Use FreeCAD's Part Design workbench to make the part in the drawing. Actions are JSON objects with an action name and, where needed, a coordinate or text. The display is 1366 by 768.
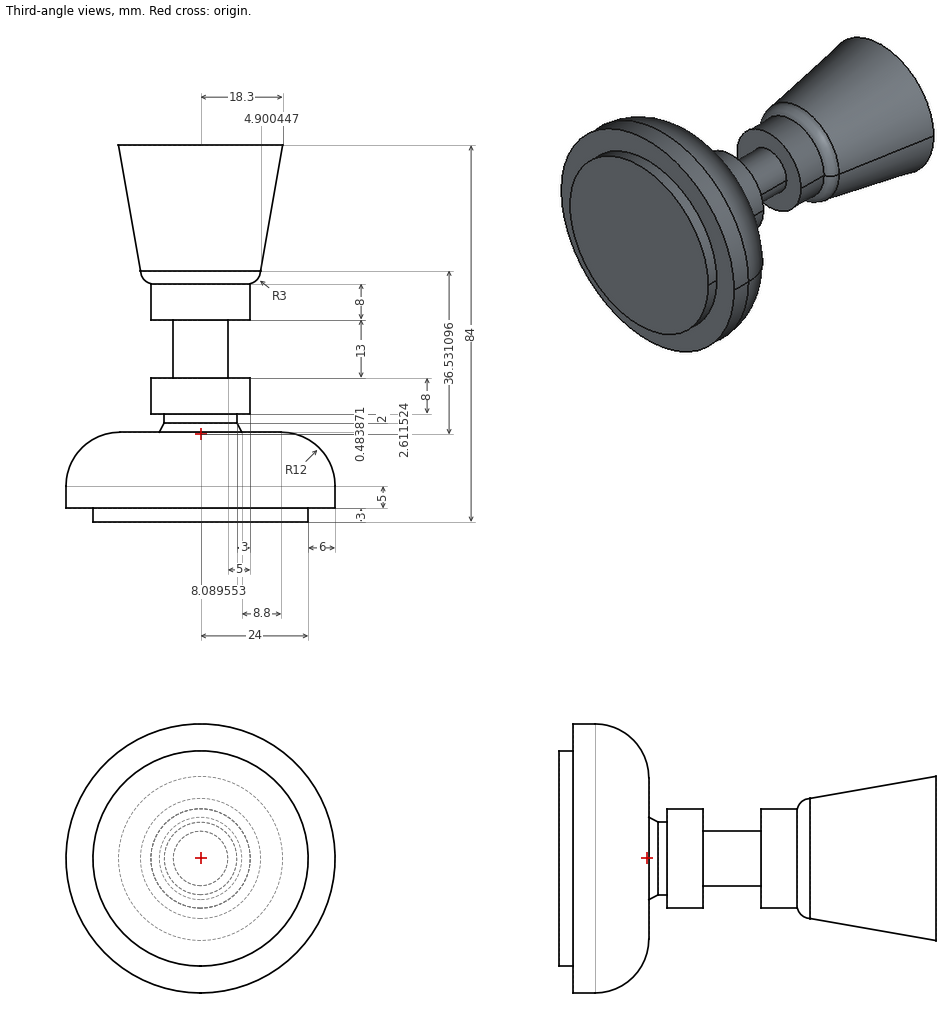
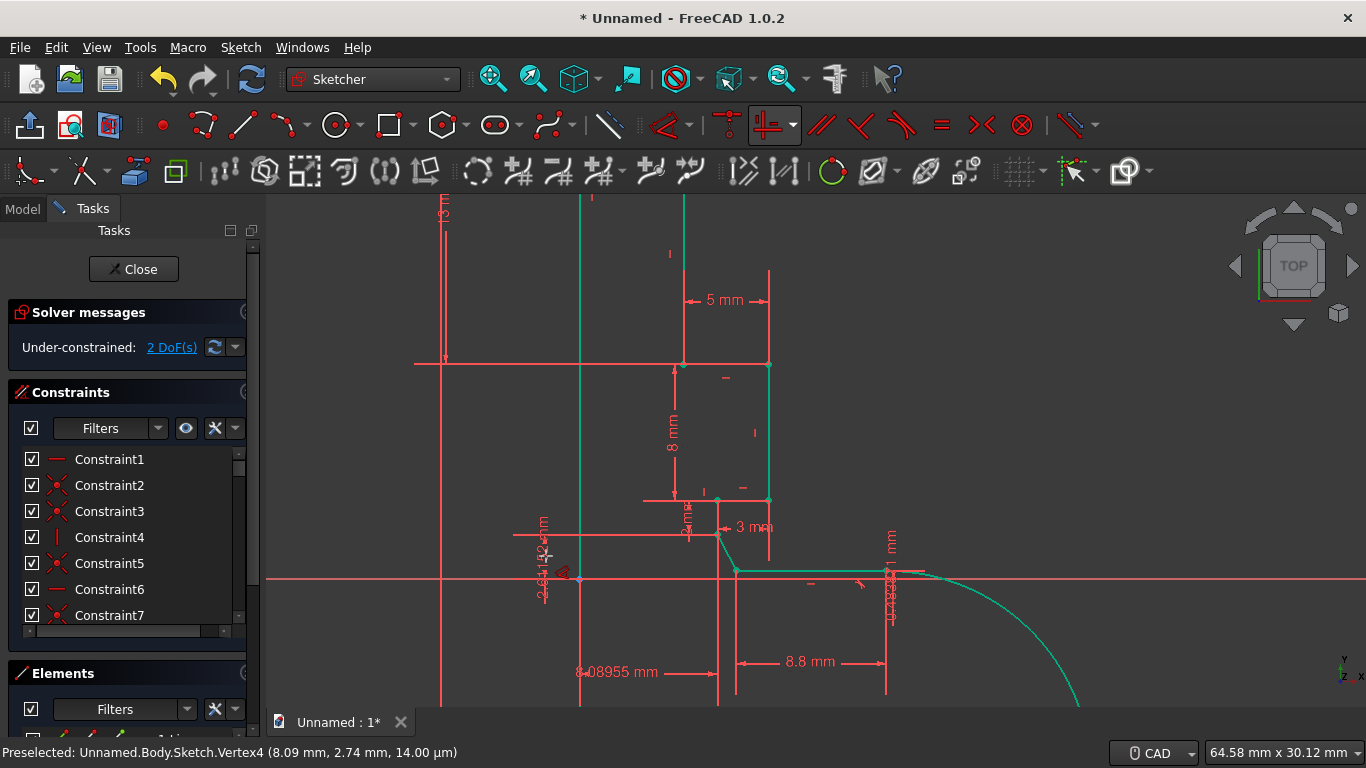
{"action": "scroll", "coordinate": [719, 534], "scroll_direction": "down", "scroll_amount": 7}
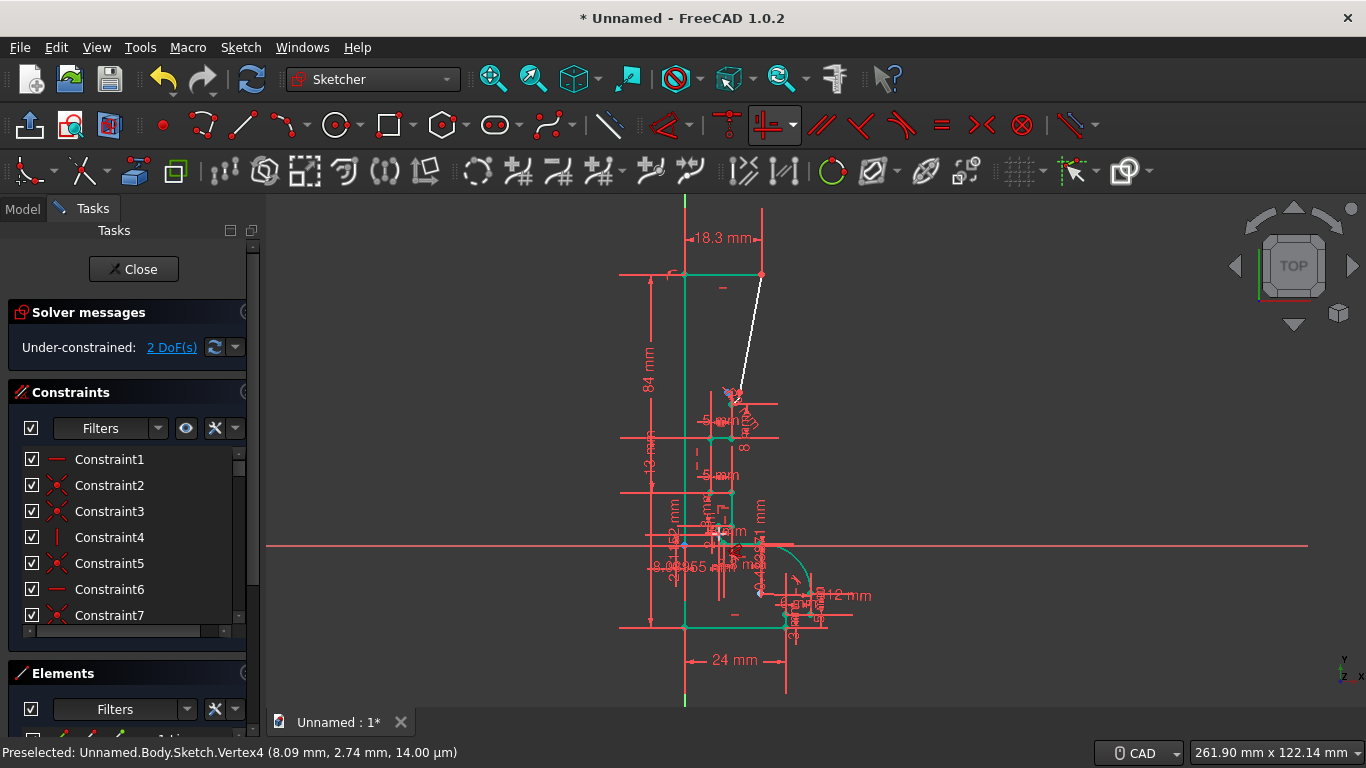
{"action": "scroll", "coordinate": [747, 357], "scroll_direction": "up", "scroll_amount": 4}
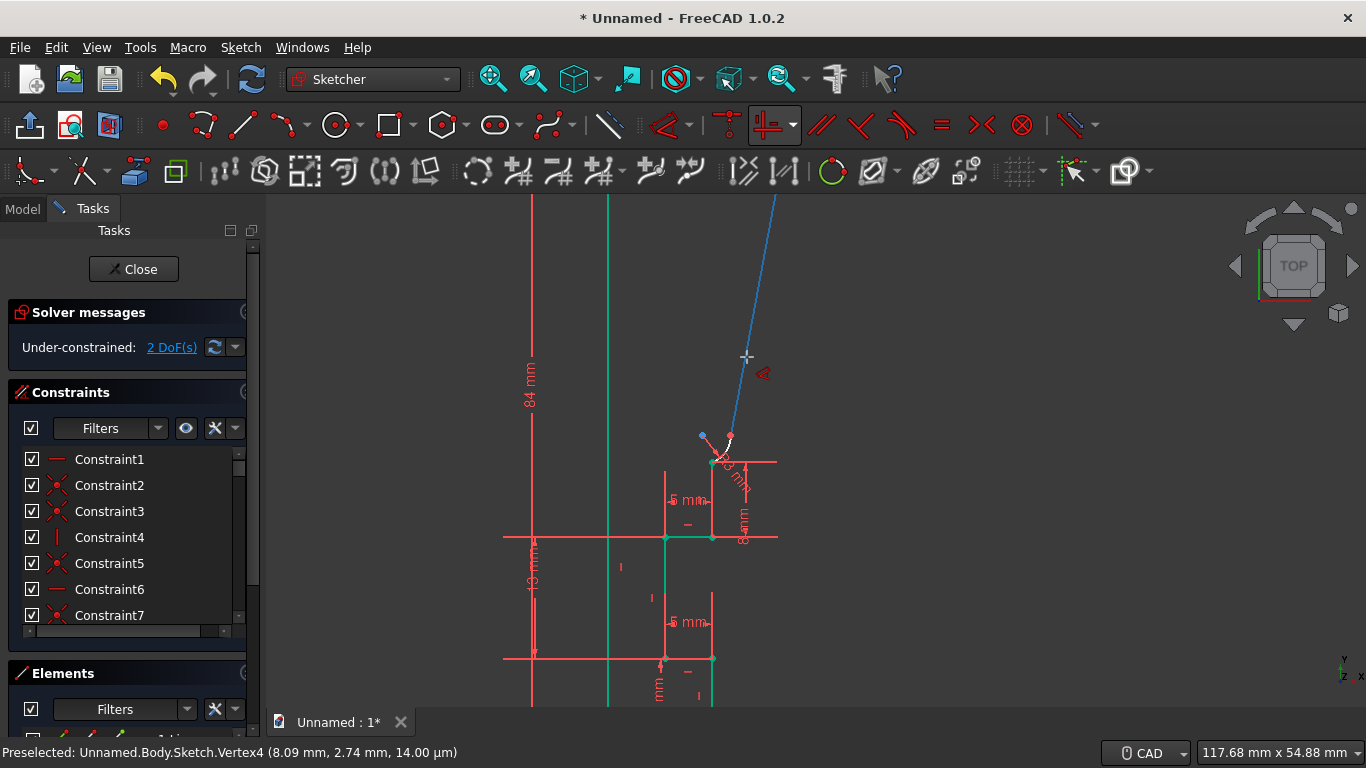
{"action": "left_click", "coordinate": [745, 357]}
{"action": "left_click", "coordinate": [755, 566]}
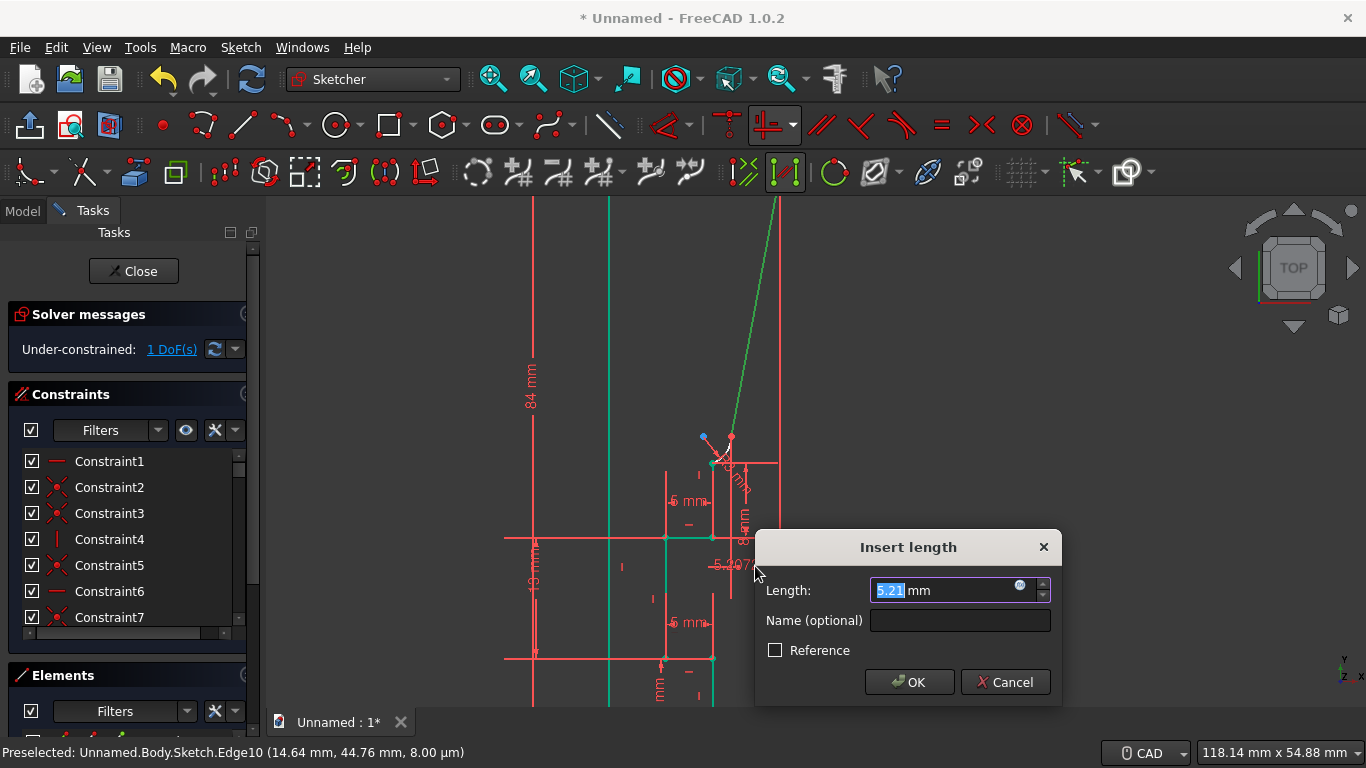
{"action": "type", "text": "4.900447"}
{"action": "key", "text": "Return"}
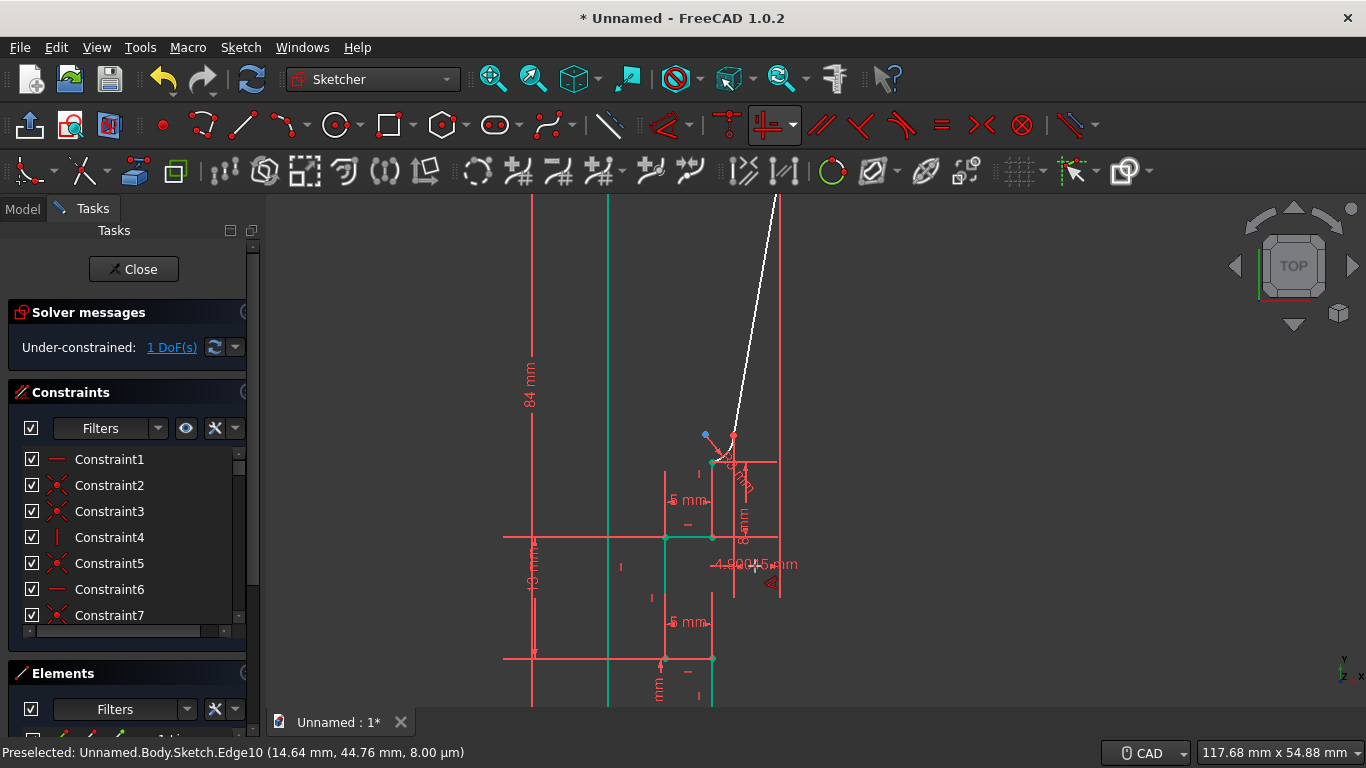
{"action": "left_click", "coordinate": [734, 436]}
{"action": "left_click", "coordinate": [574, 501]}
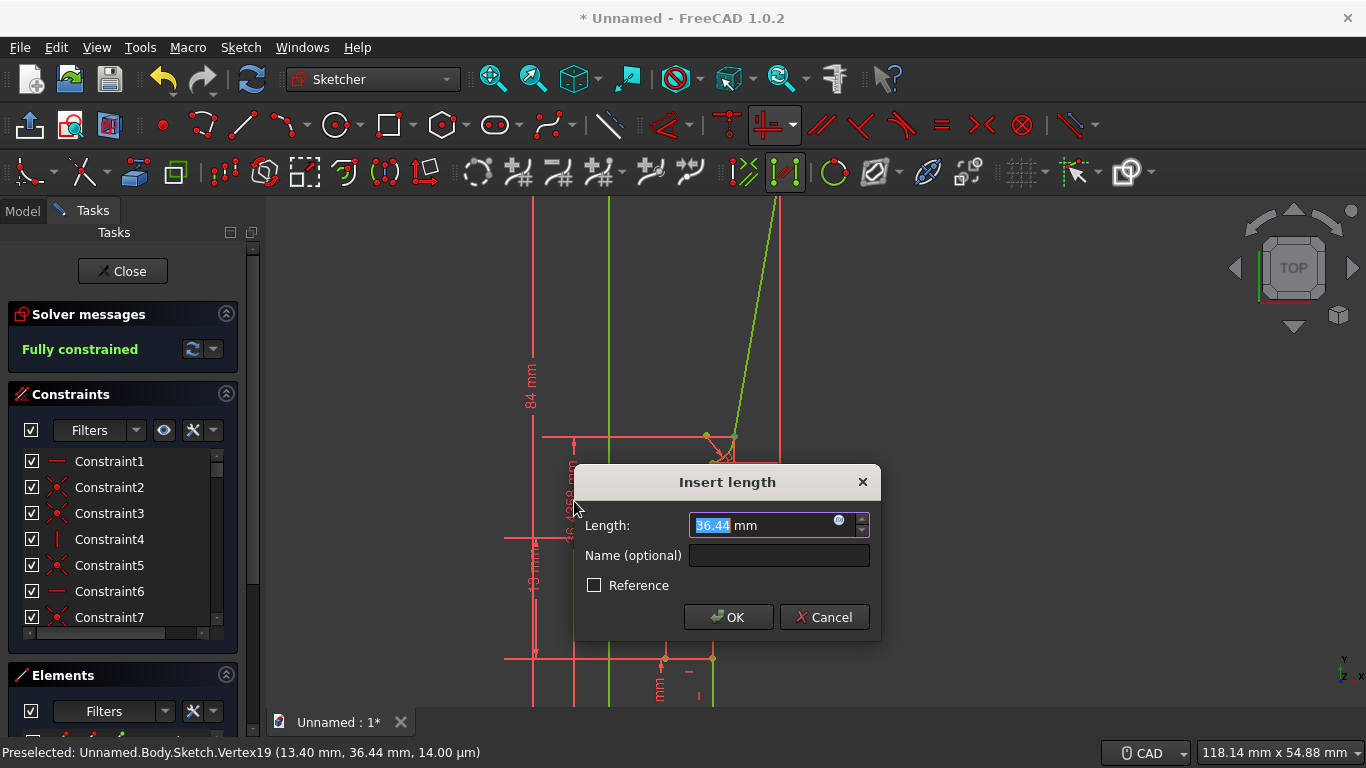
{"action": "type", "text": "36.531096"}
{"action": "key", "text": "Return"}
{"action": "key", "text": "Escape"}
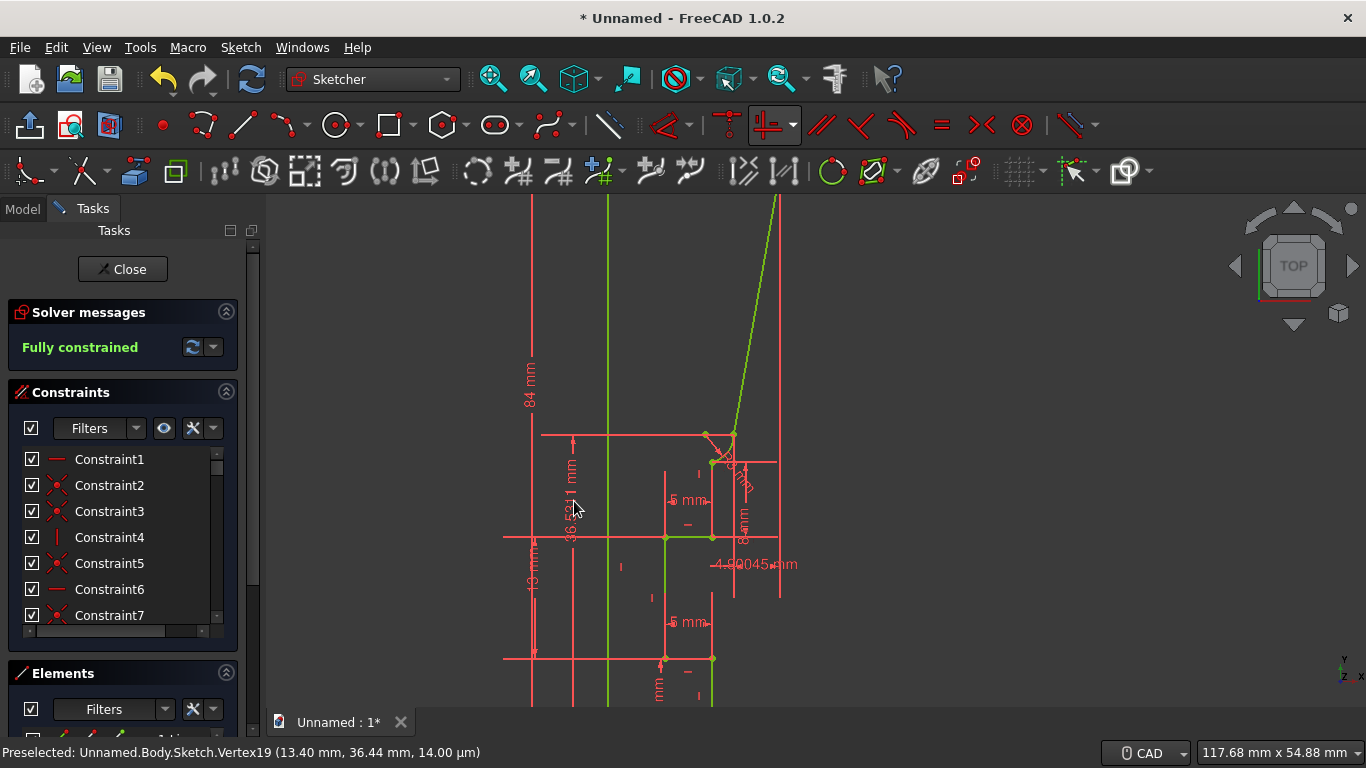
{"action": "left_click", "coordinate": [123, 269]}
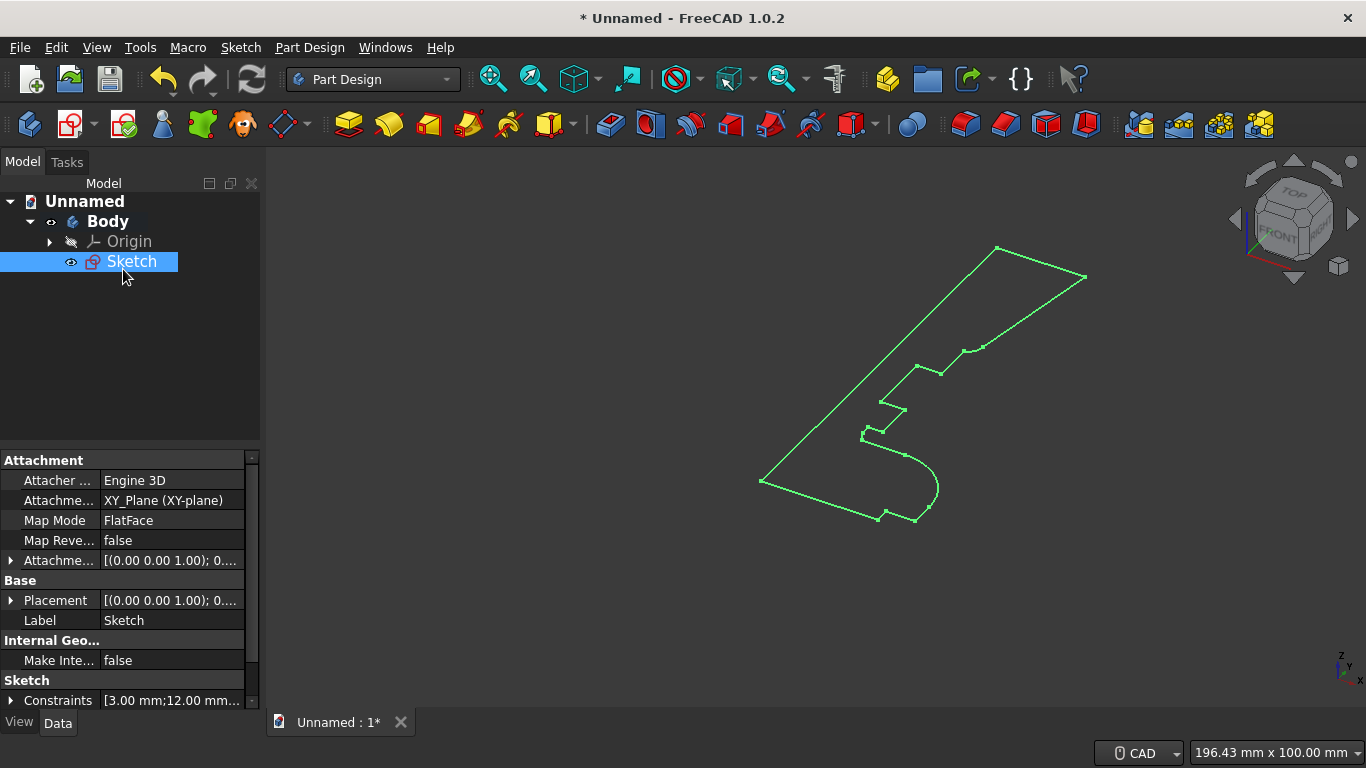
{"action": "left_click", "coordinate": [390, 124]}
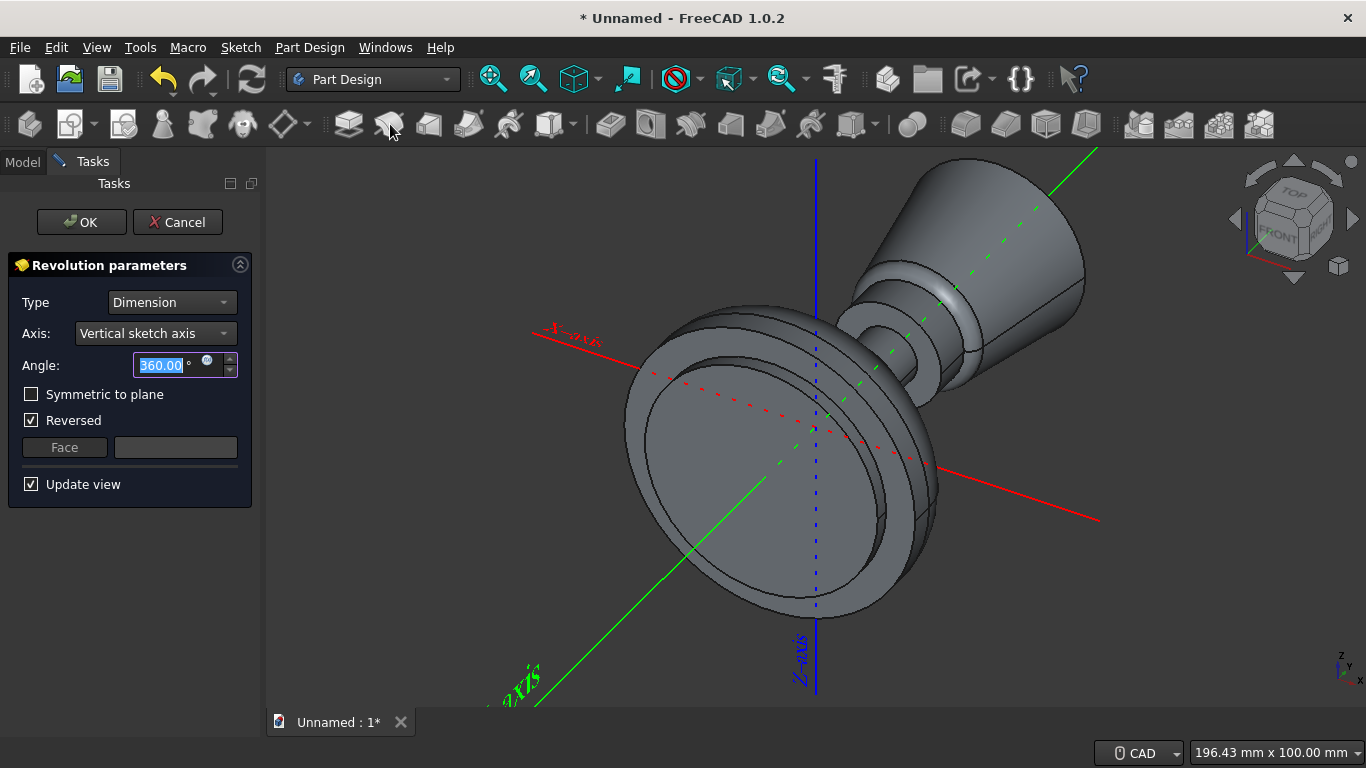
{"action": "left_click", "coordinate": [82, 222]}